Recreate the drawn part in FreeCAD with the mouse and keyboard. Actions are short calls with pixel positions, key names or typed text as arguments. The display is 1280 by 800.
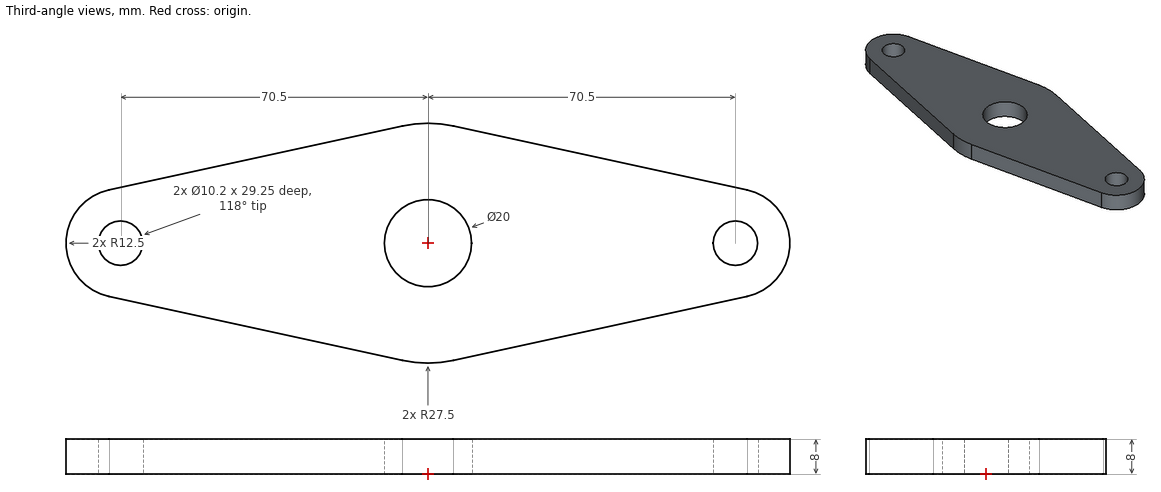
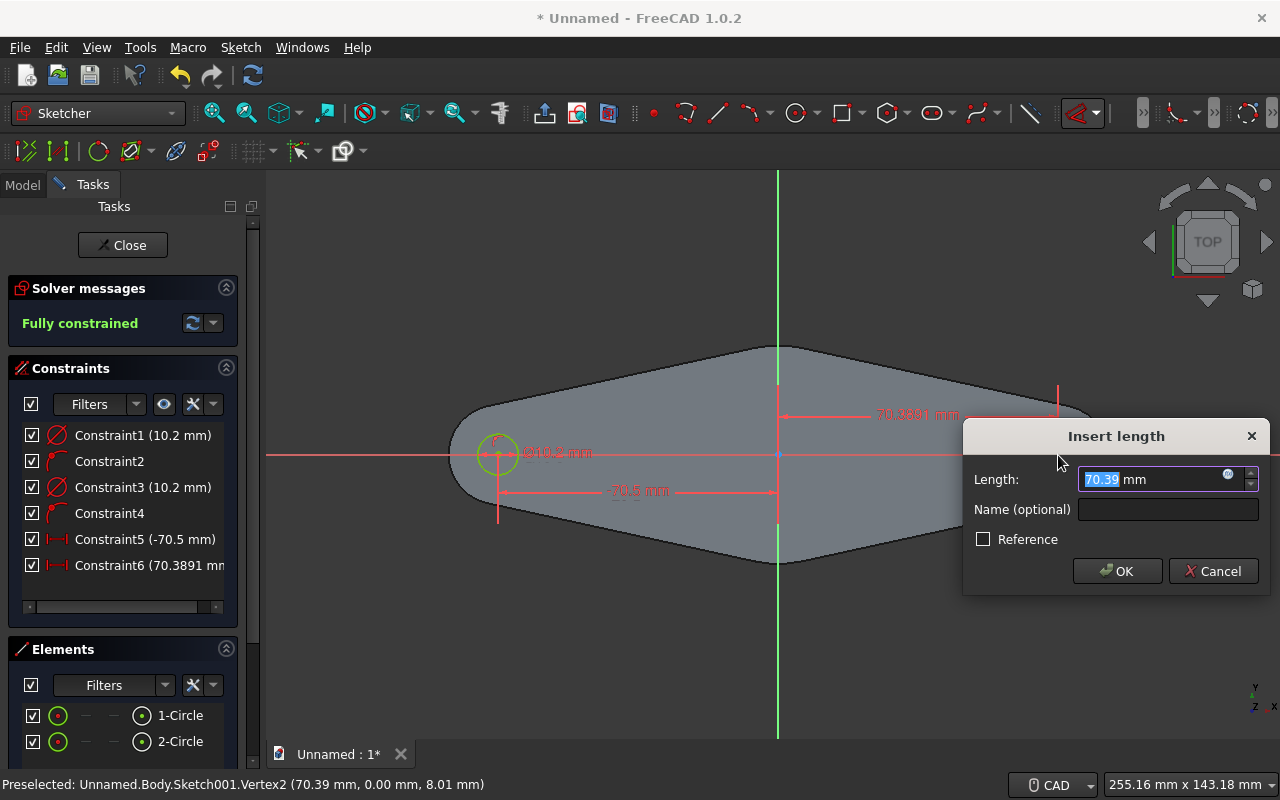
text(70.5)
key(Return)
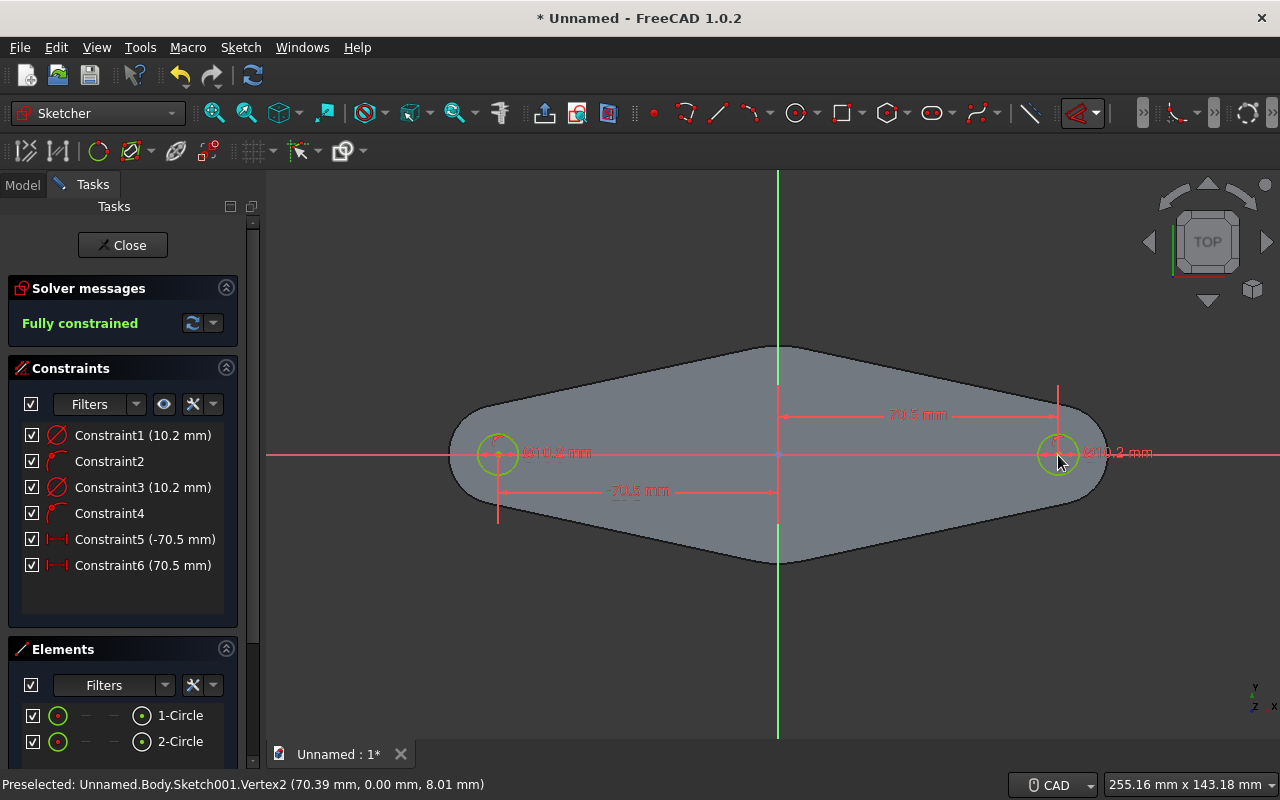
click(123, 245)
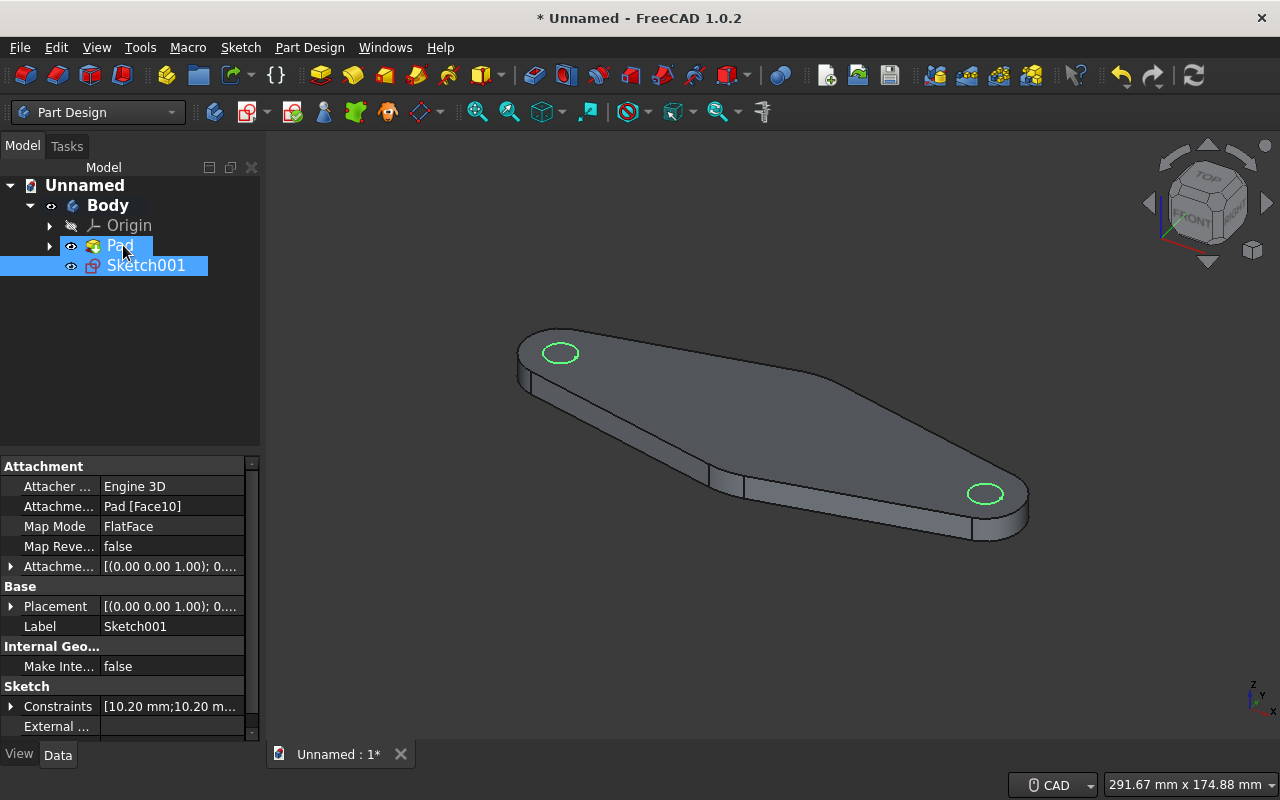
click(568, 76)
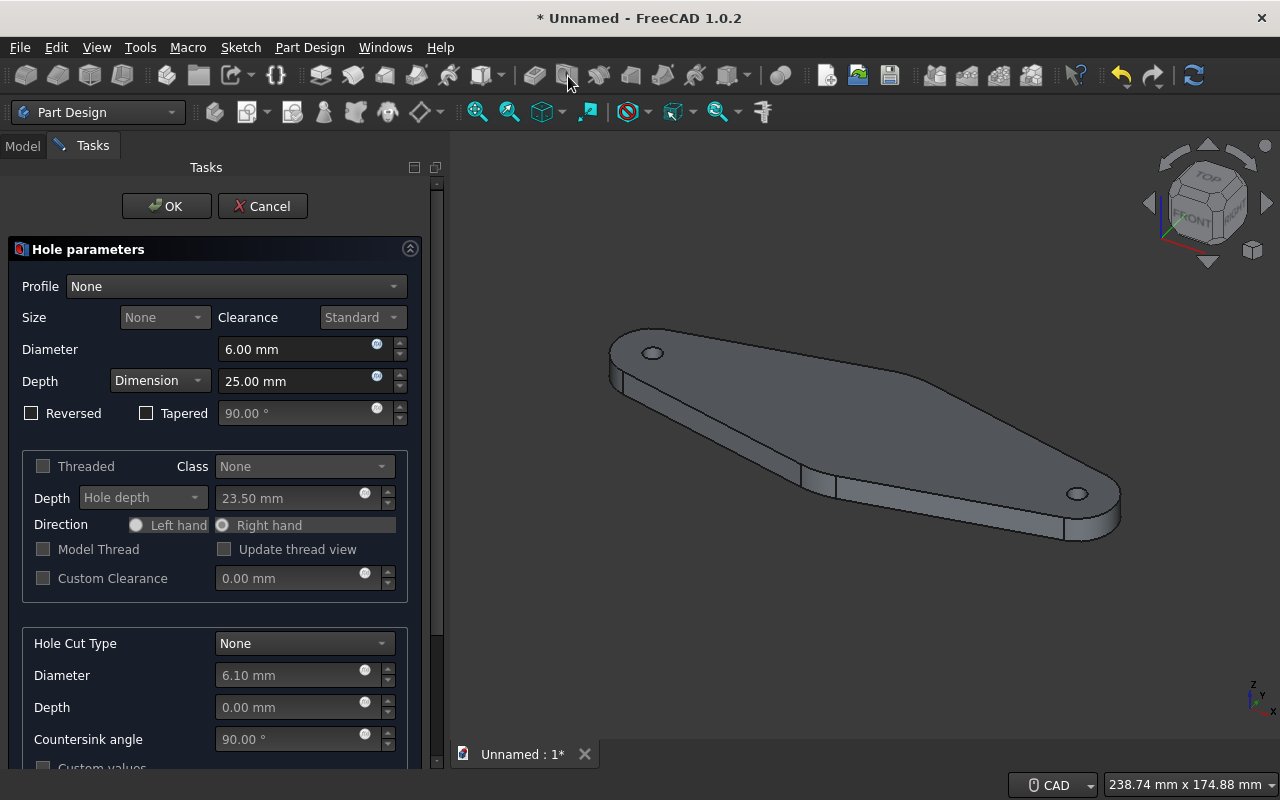
triple_click(305, 349)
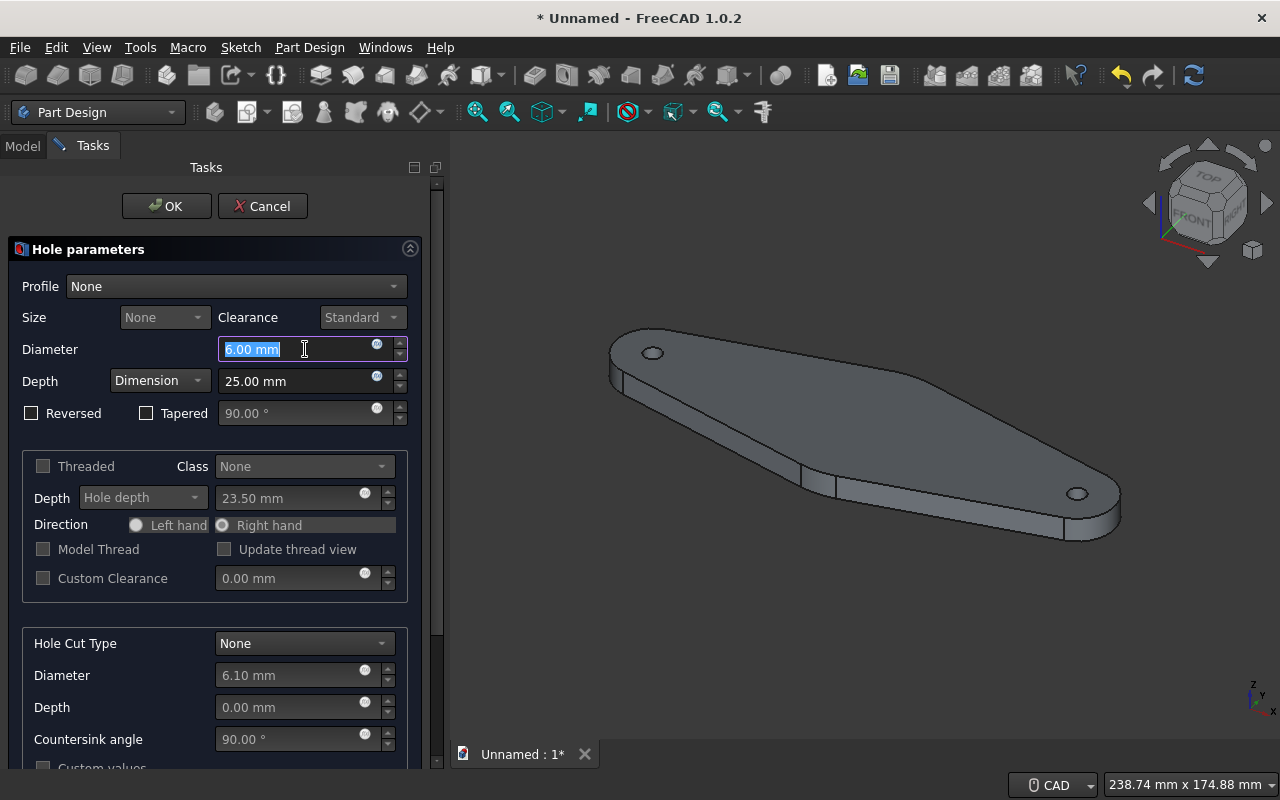
text(10.2)
key(Tab)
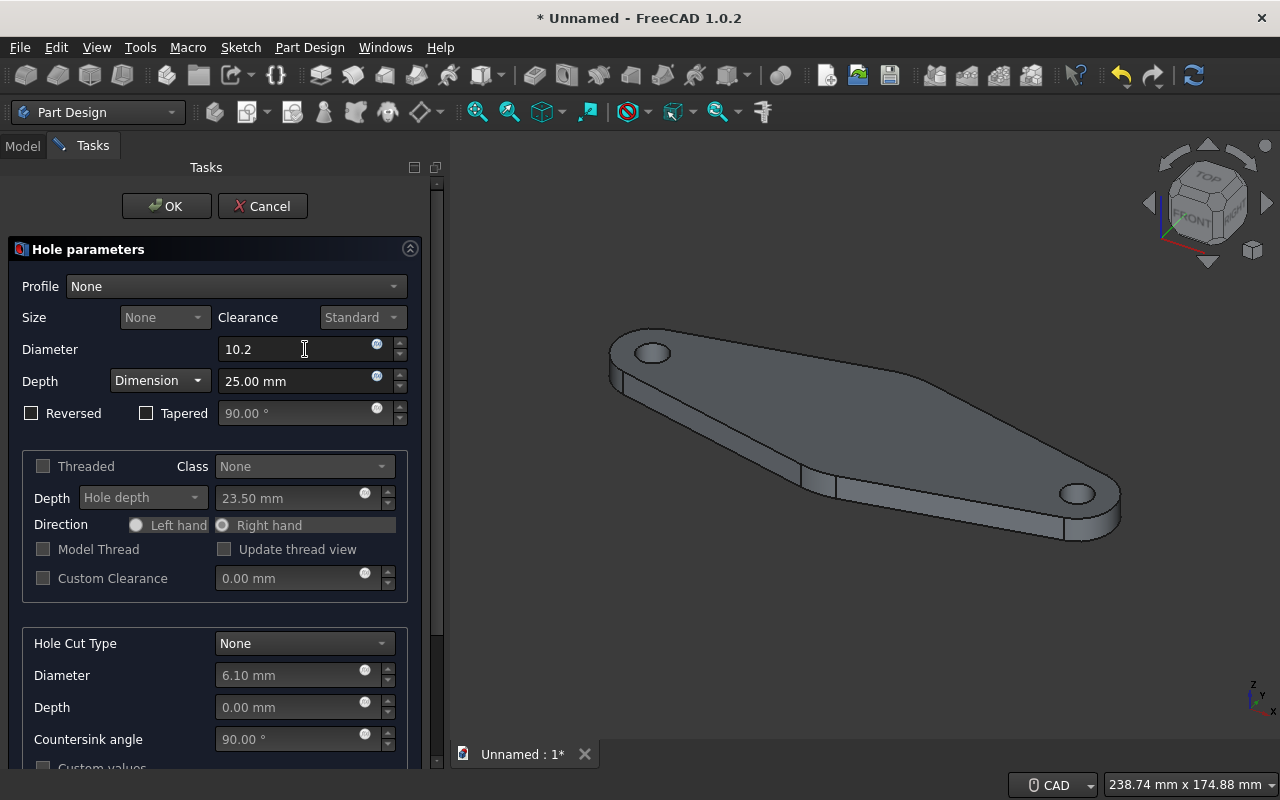
triple_click(305, 381)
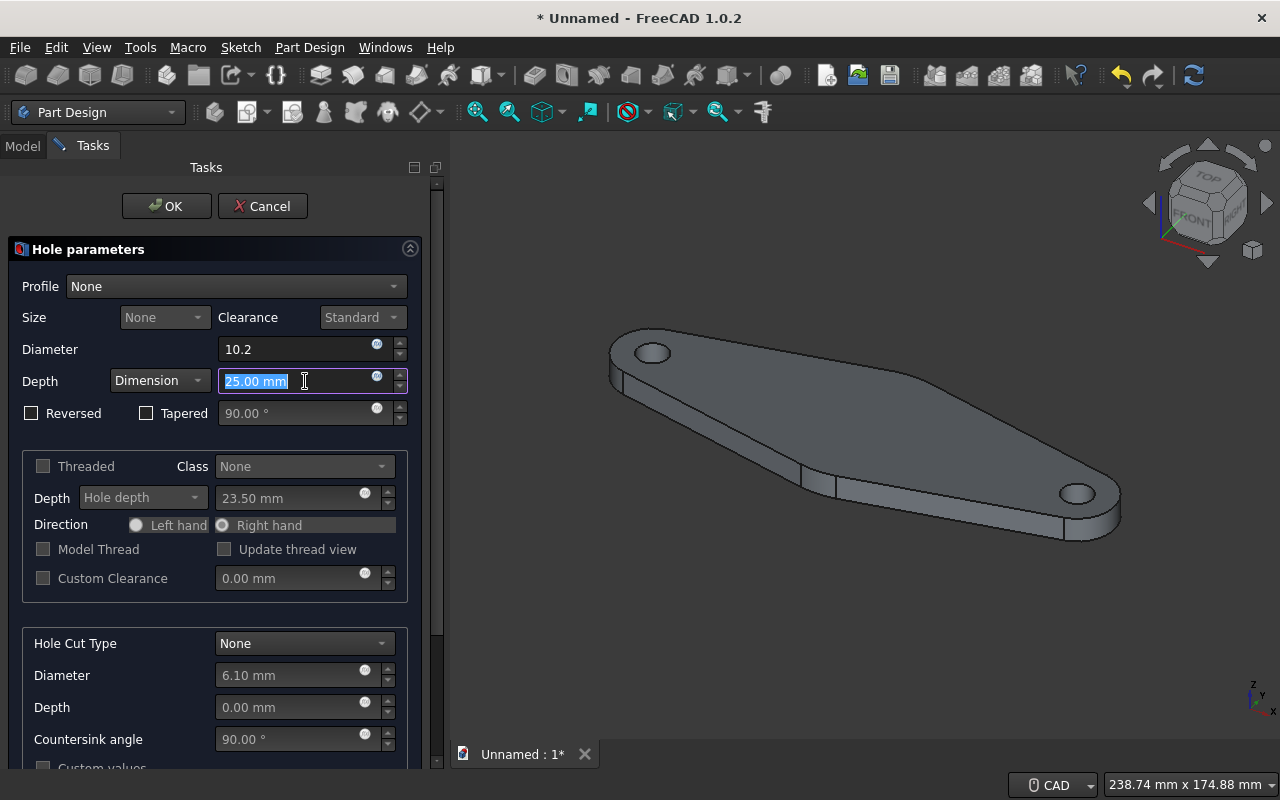
text(29.25)
key(Tab)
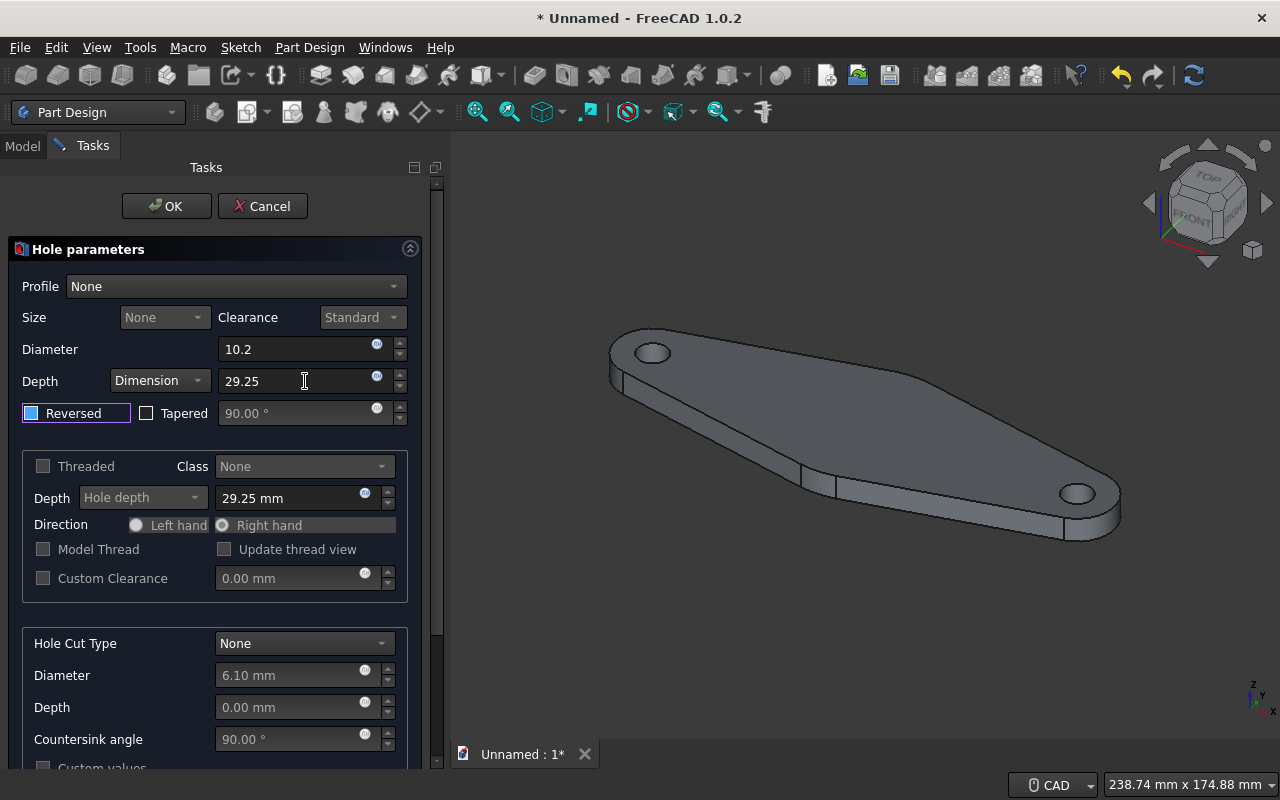
click(167, 206)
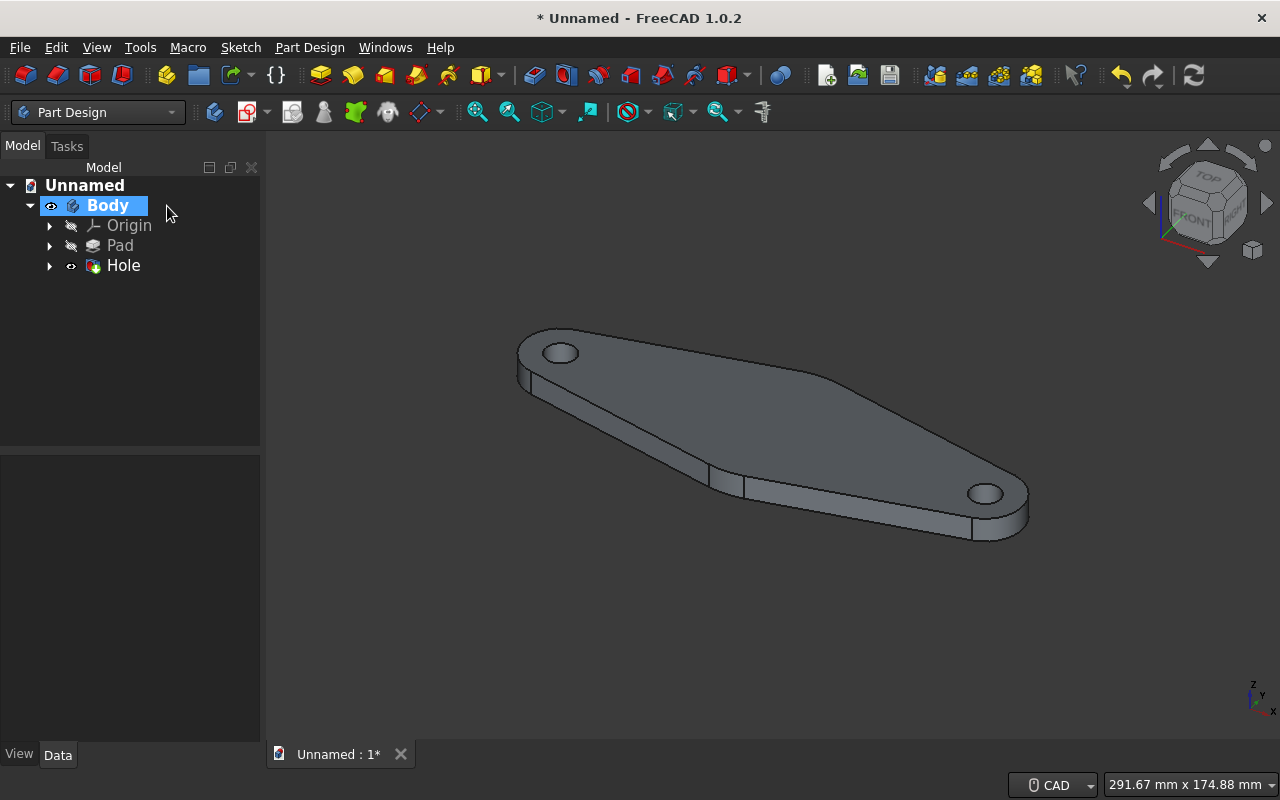
click(773, 423)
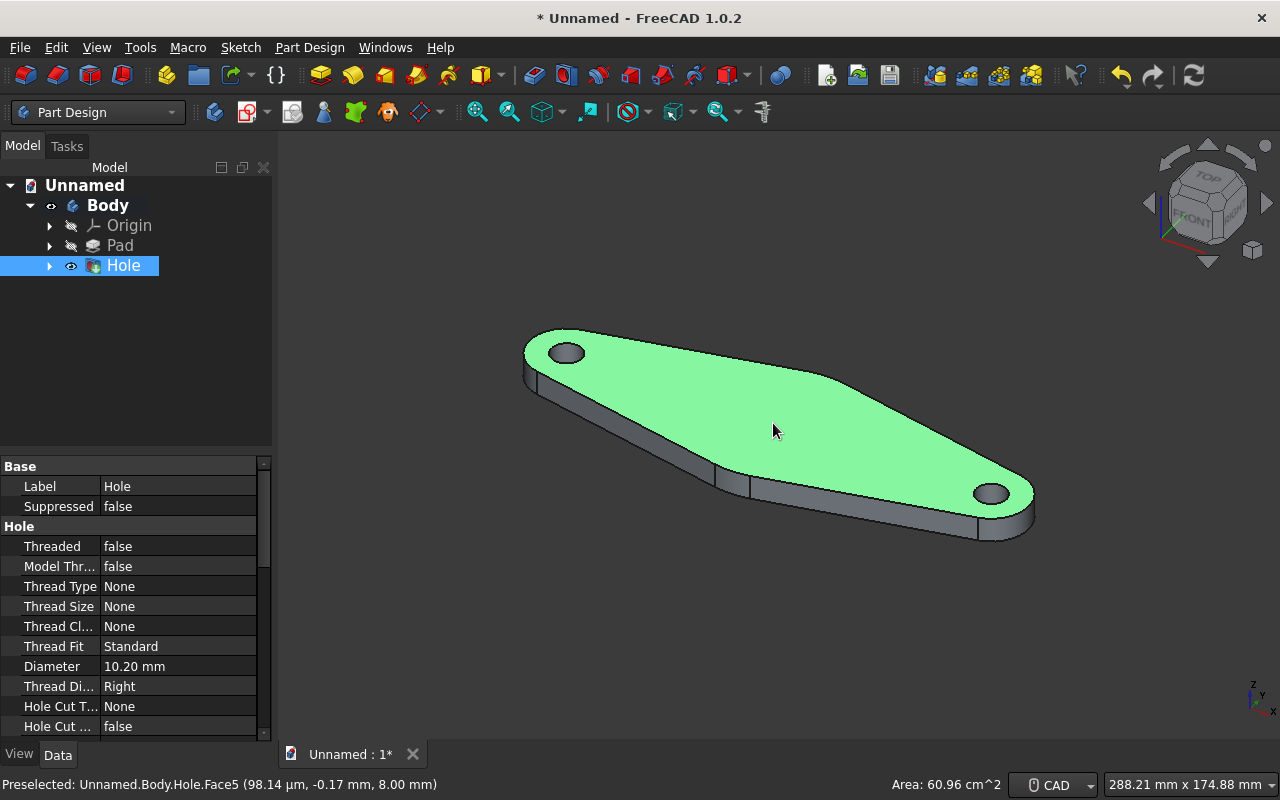
click(248, 112)